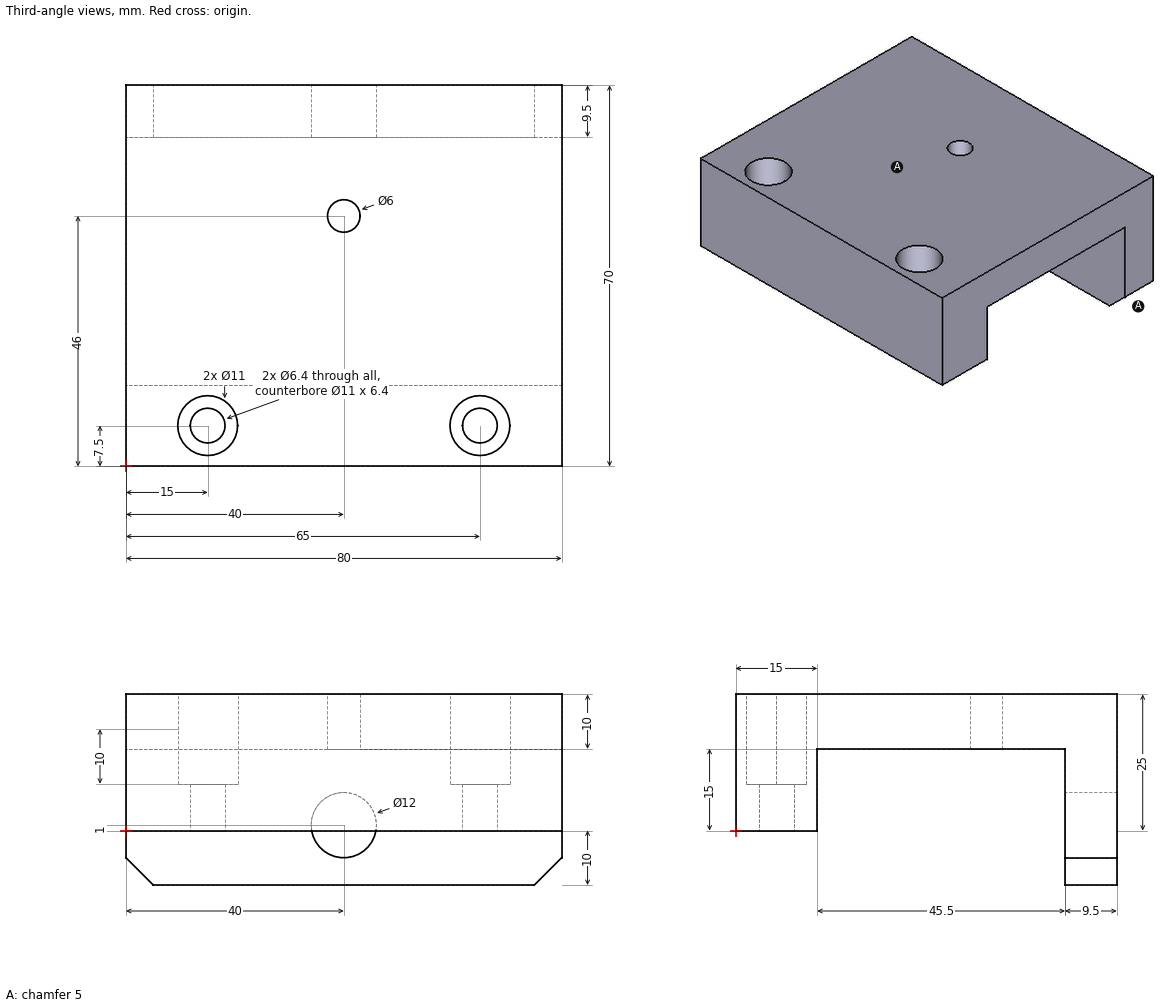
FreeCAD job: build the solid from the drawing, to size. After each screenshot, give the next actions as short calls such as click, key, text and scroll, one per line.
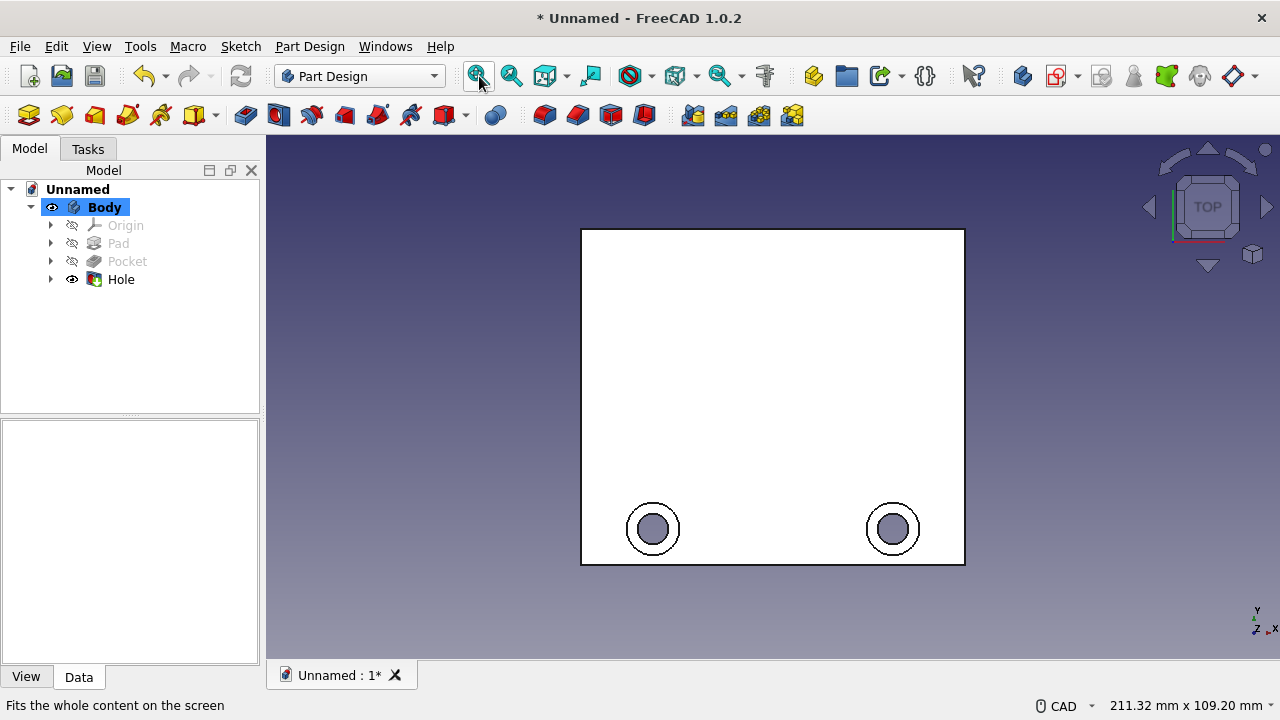
scroll(908, 543, up, 5)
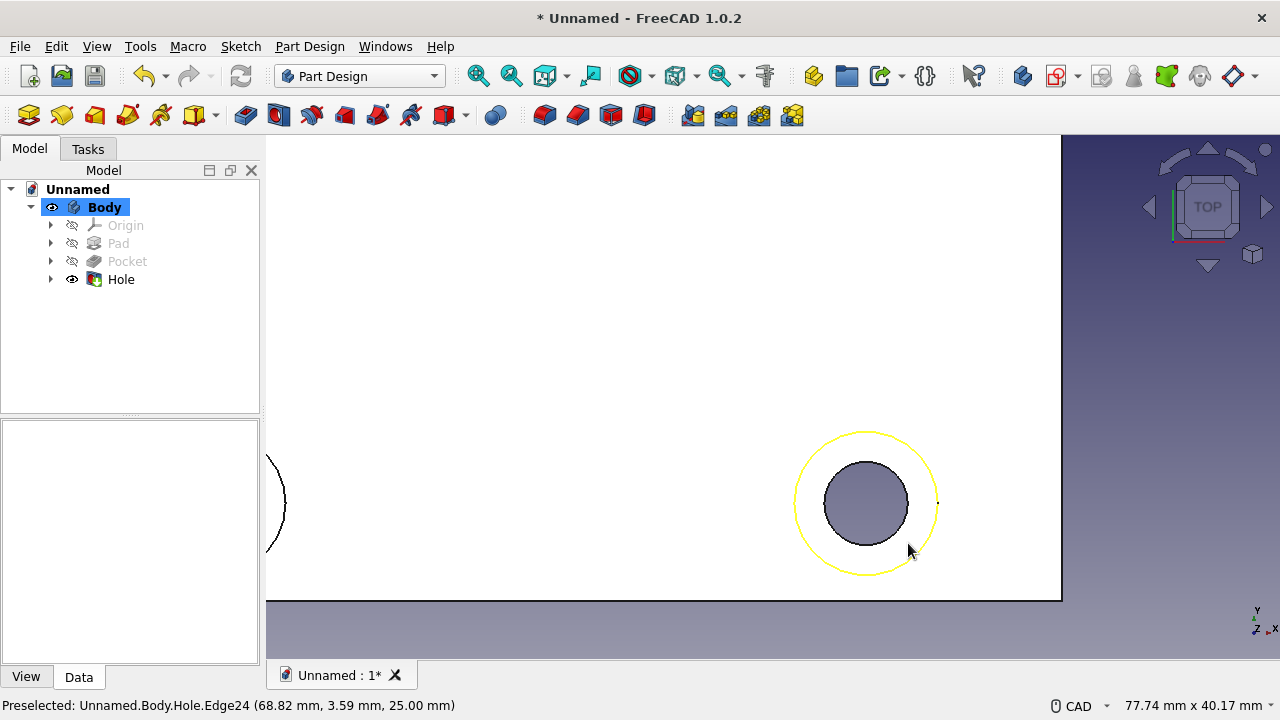
click(907, 543)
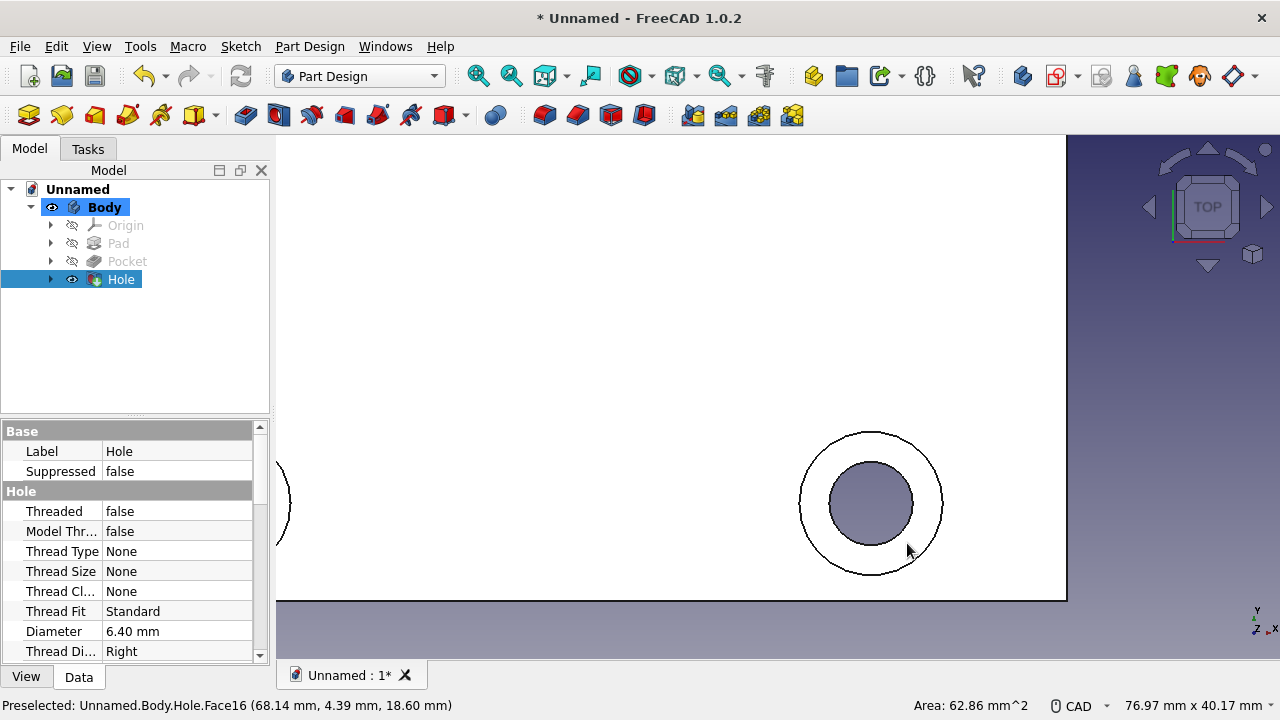
click(1056, 76)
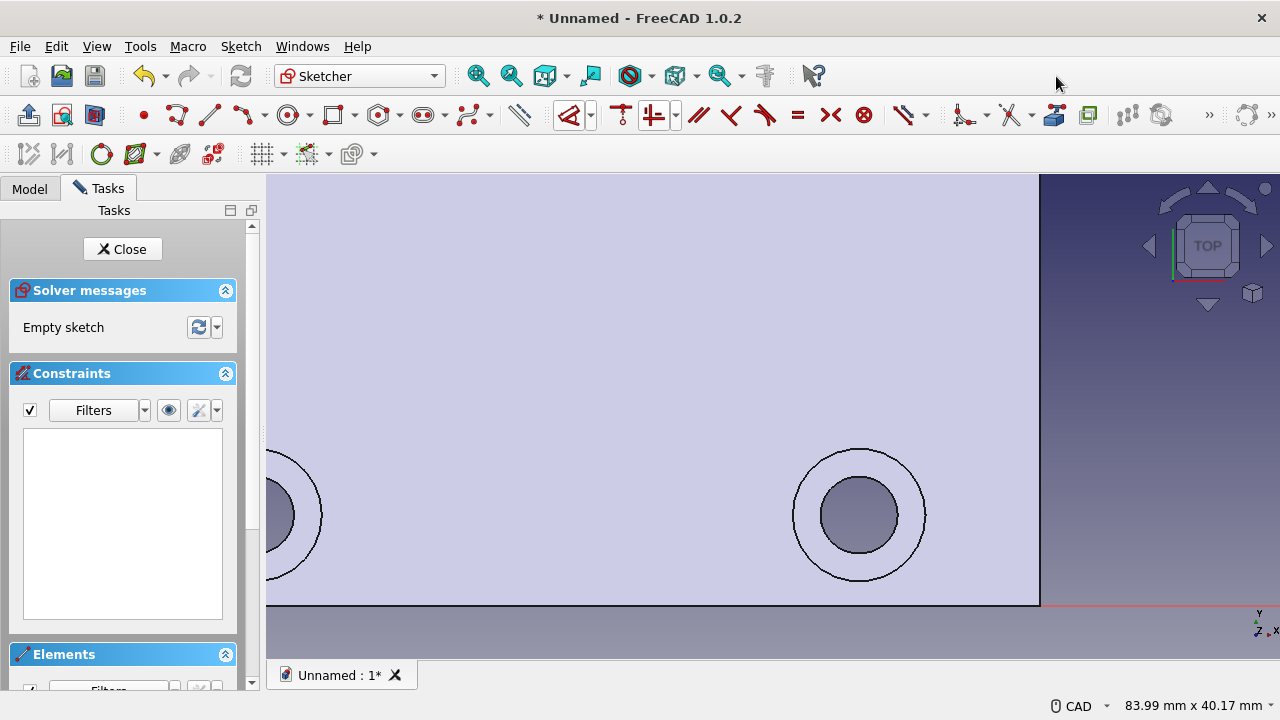
scroll(1115, 202, down, 2)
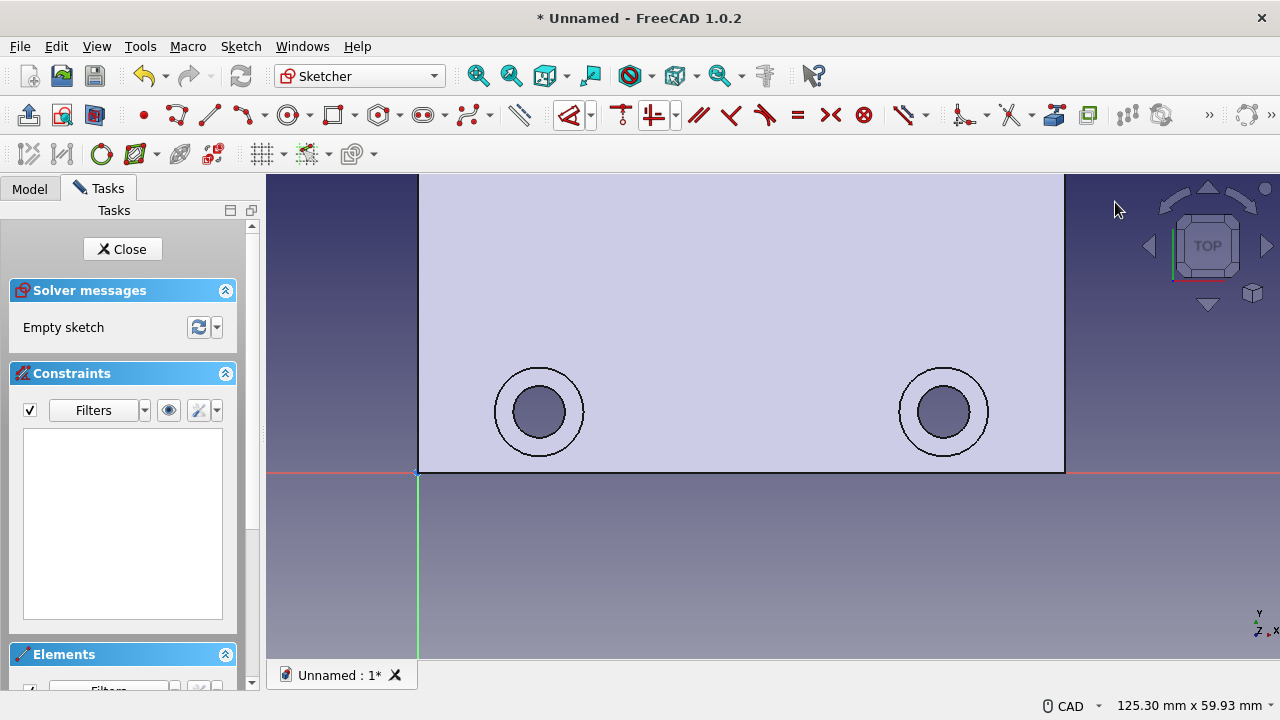
click(288, 116)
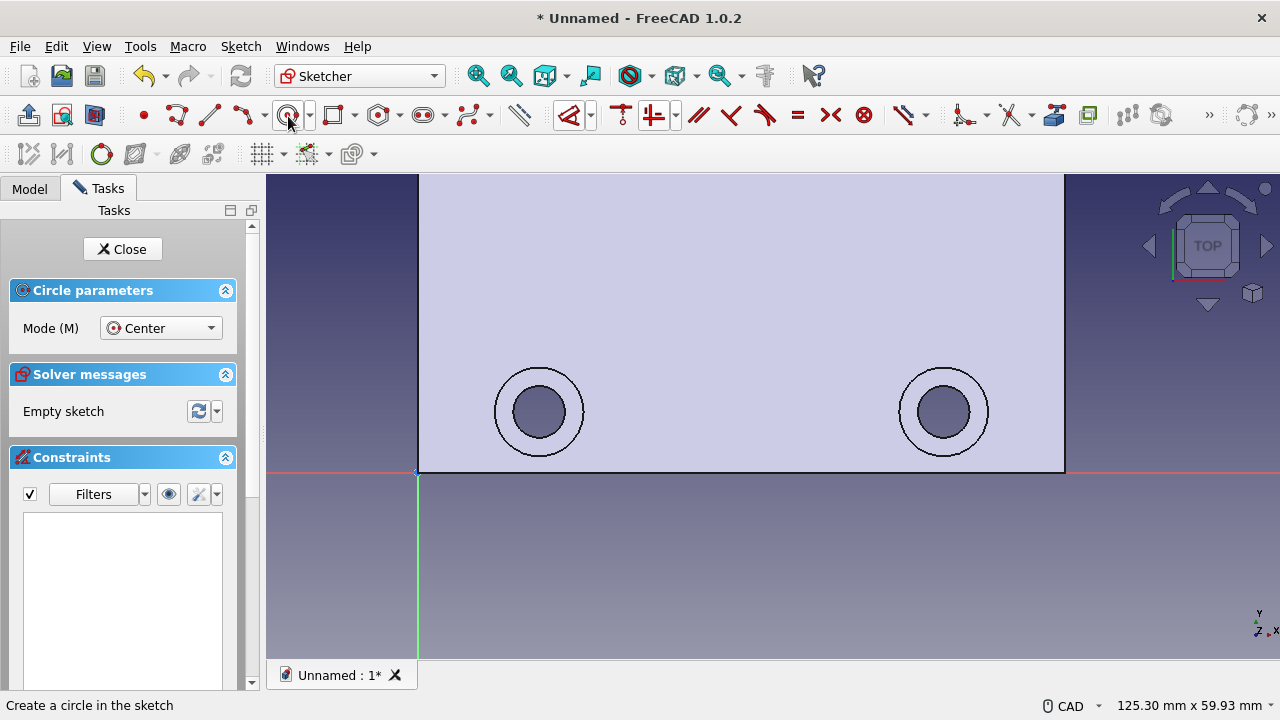
click(539, 412)
move(571, 380)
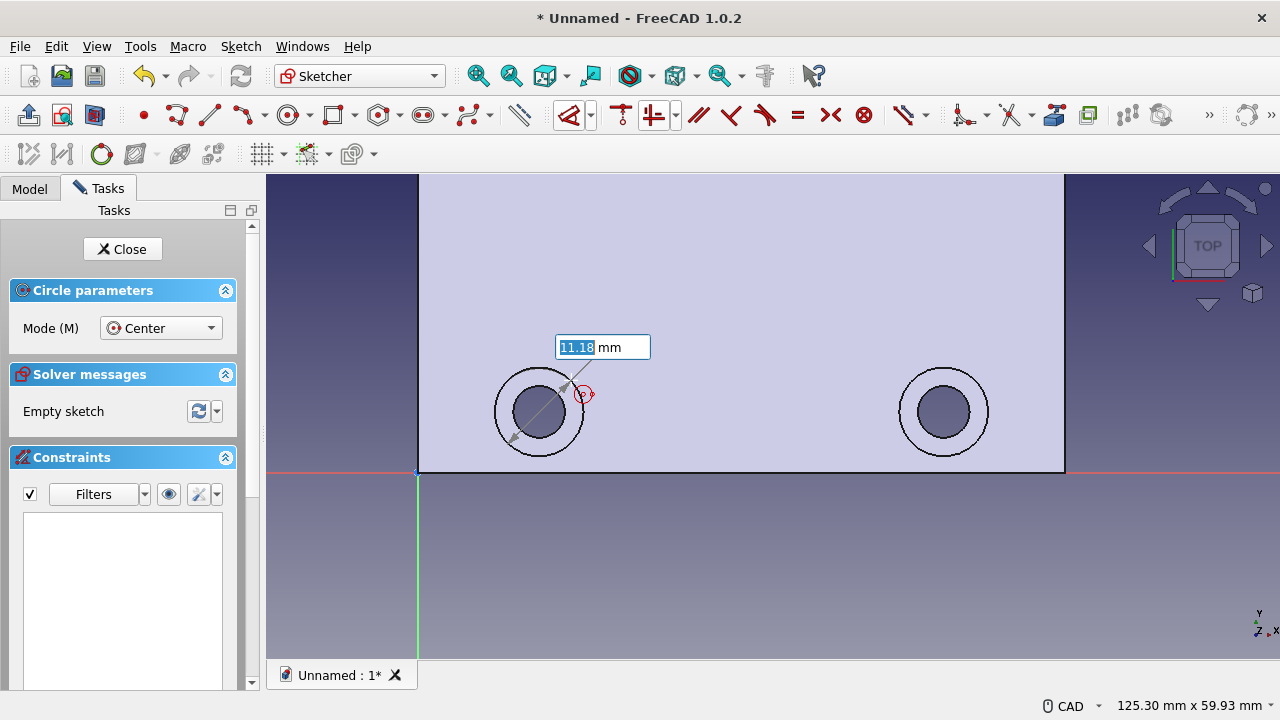
text(11)
key(Return)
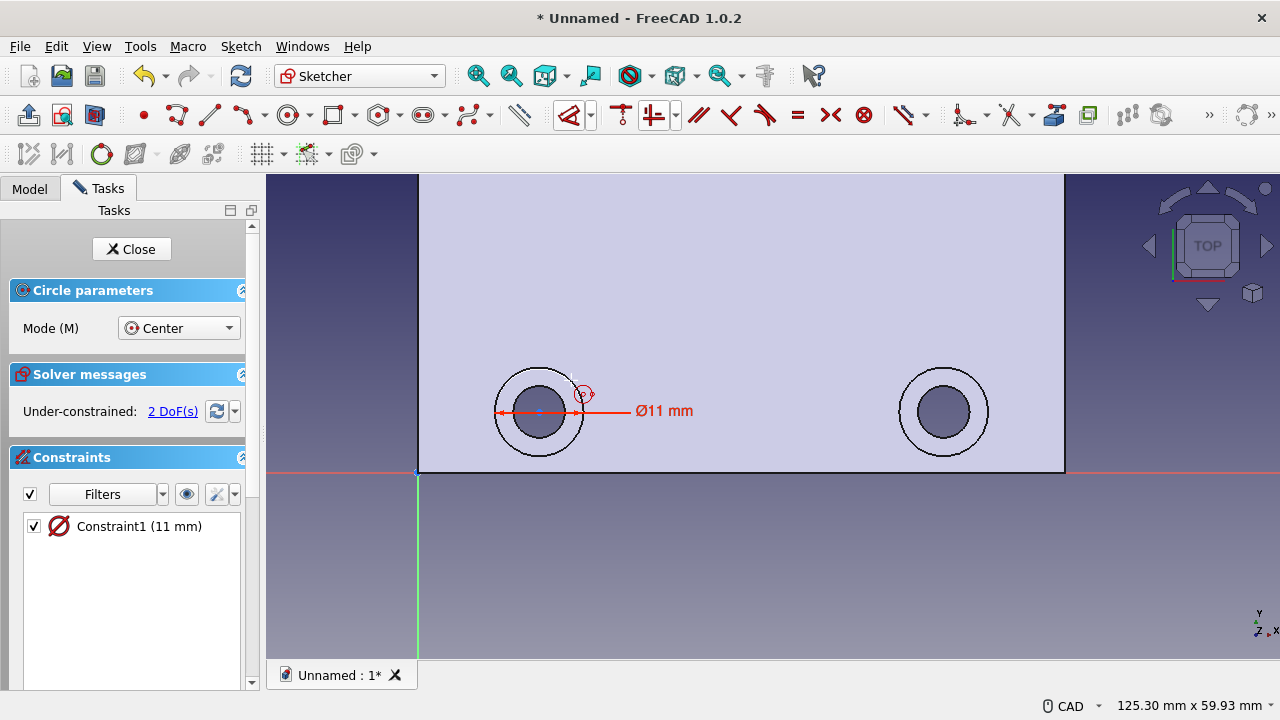
click(944, 412)
move(975, 380)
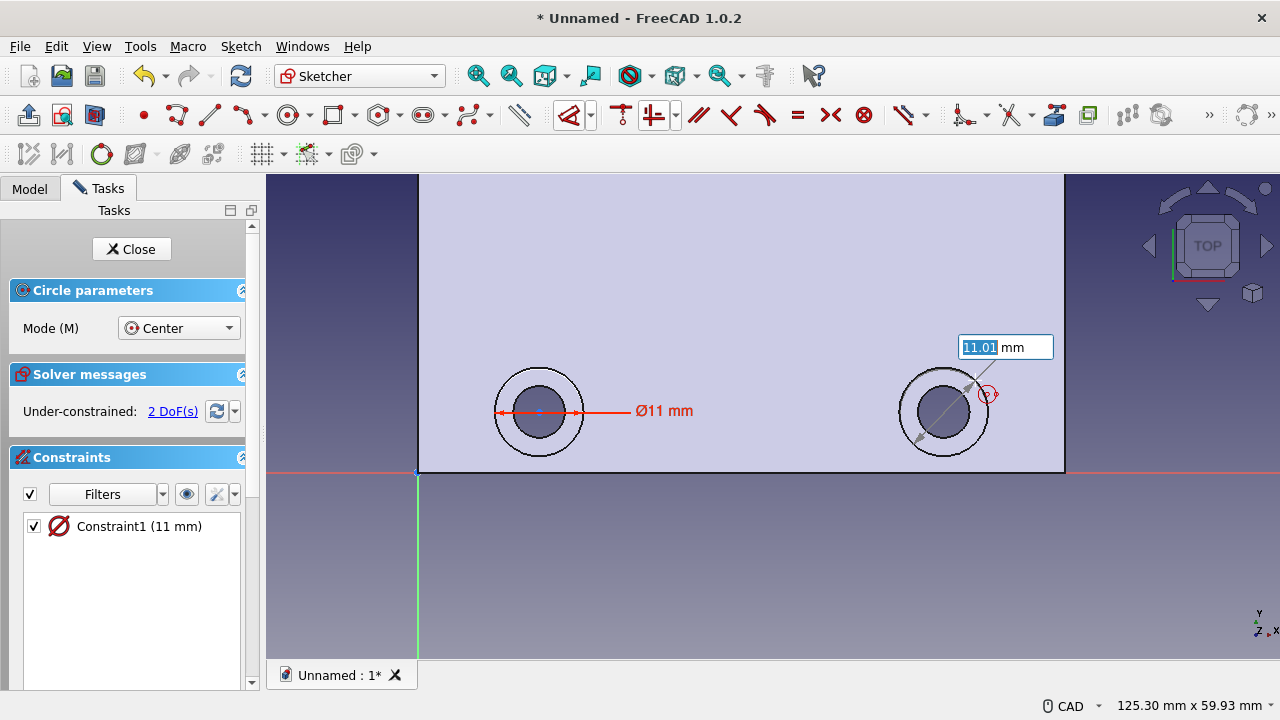
text(11)
key(Return)
key(Escape)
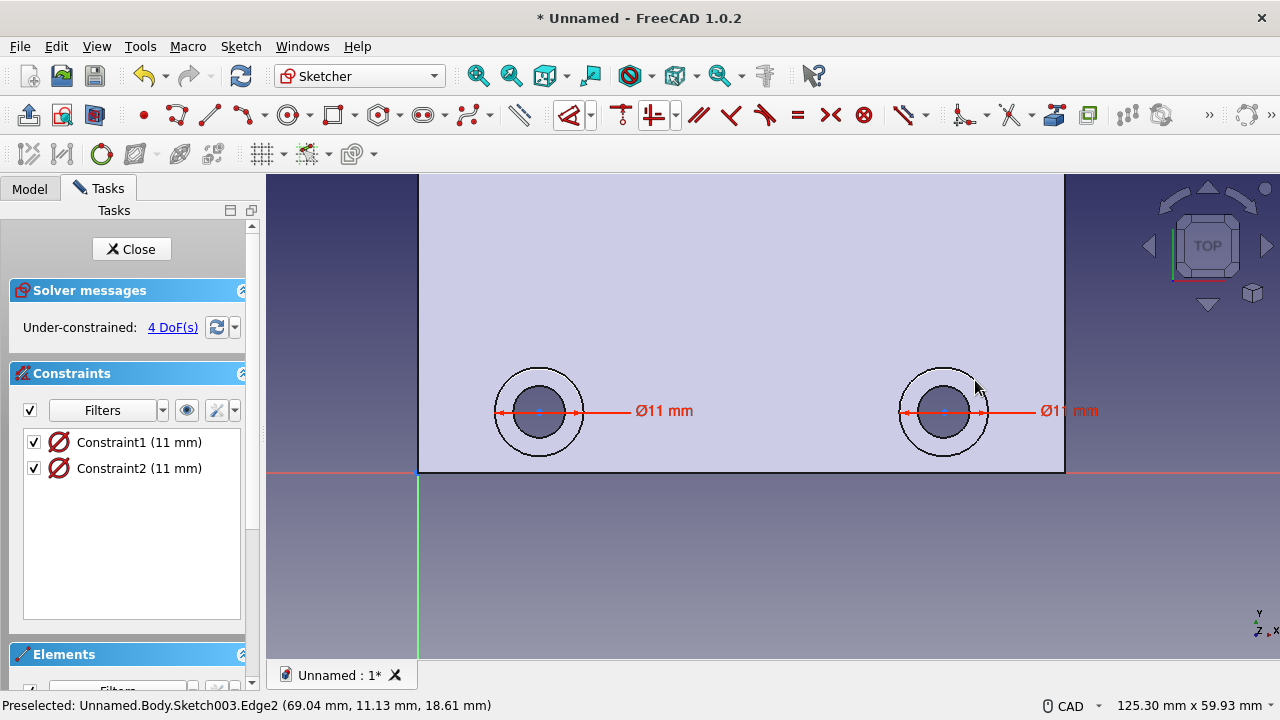
click(539, 413)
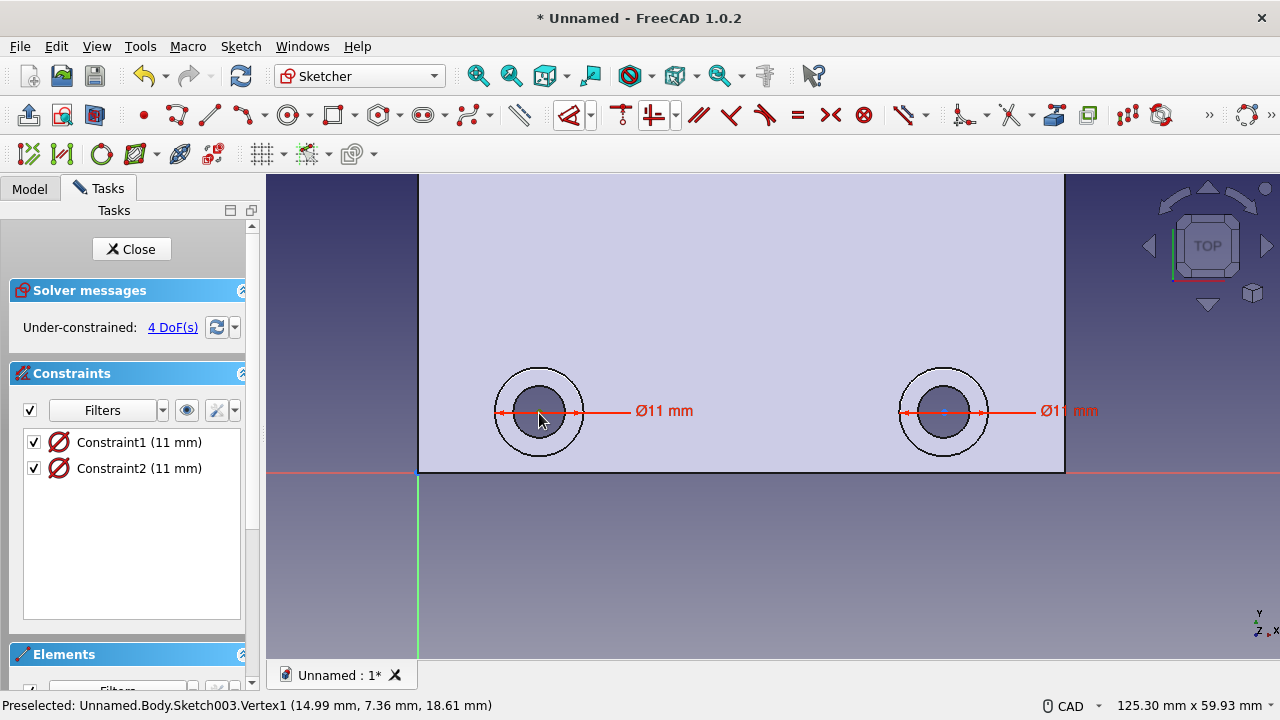
click(944, 413)